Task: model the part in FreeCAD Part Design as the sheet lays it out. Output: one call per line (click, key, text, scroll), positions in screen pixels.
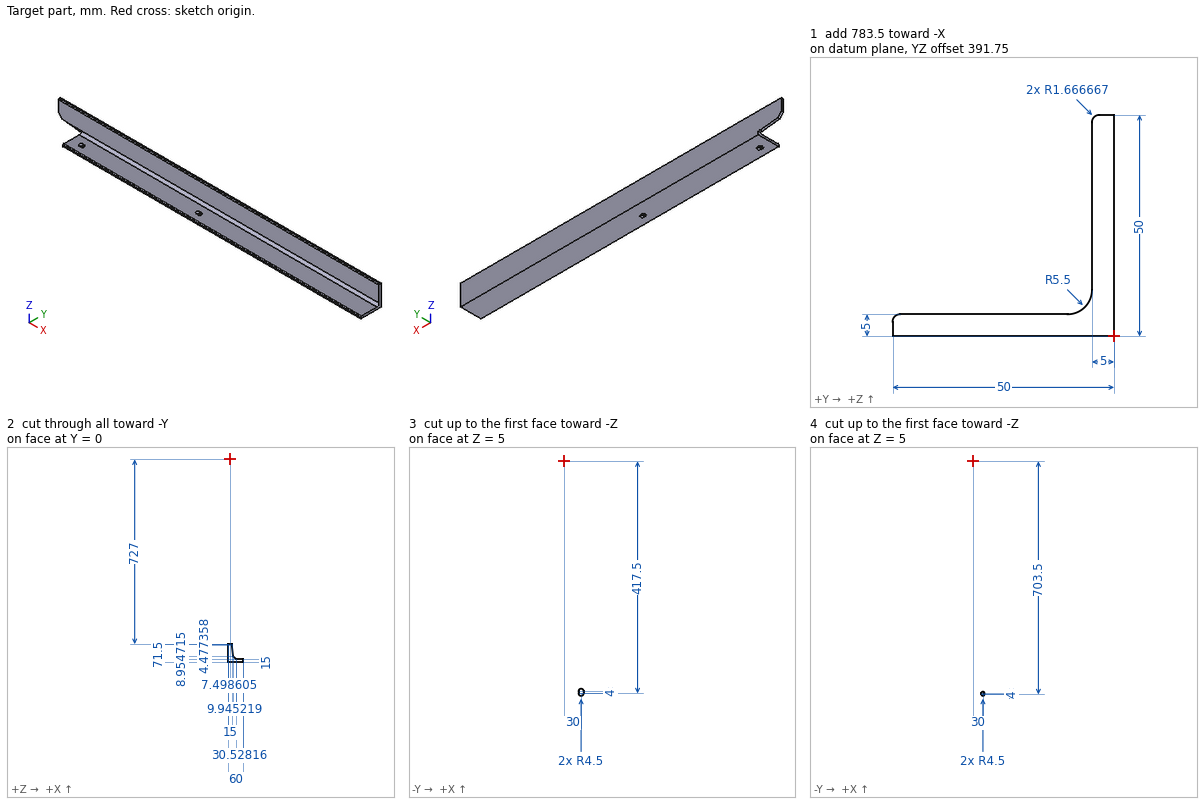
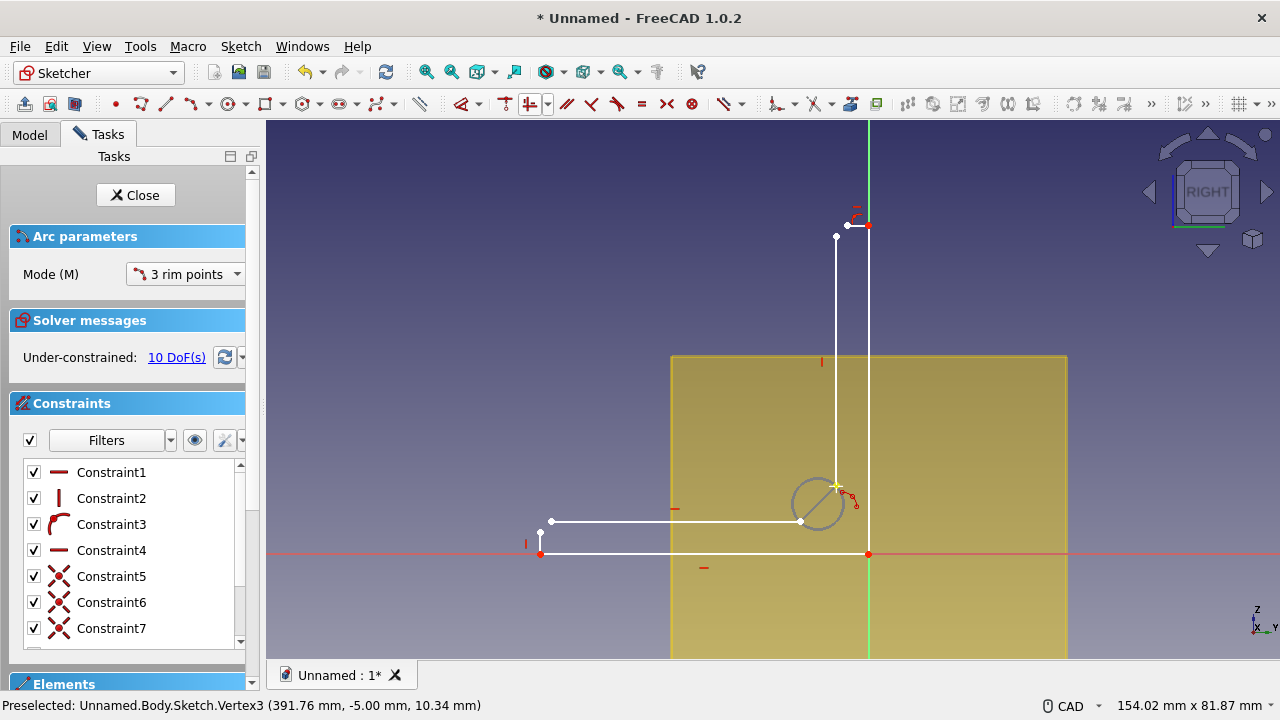
scroll(825, 511, up, 3)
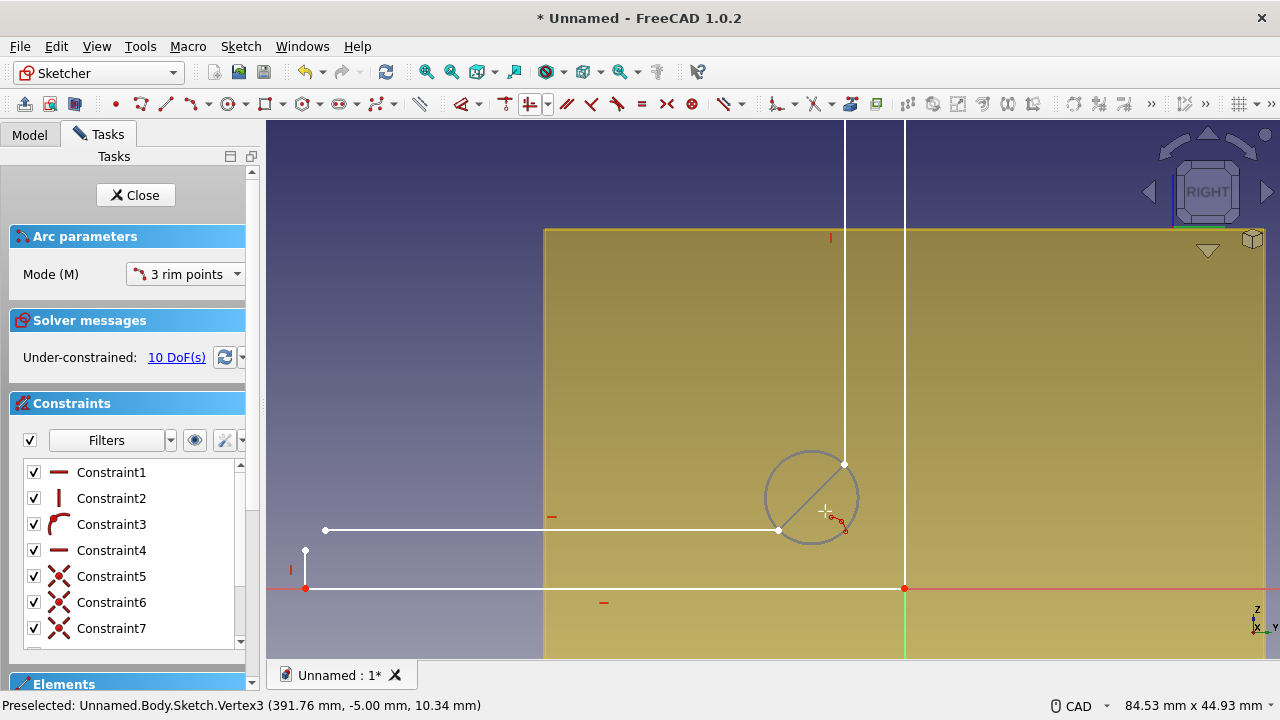
click(825, 510)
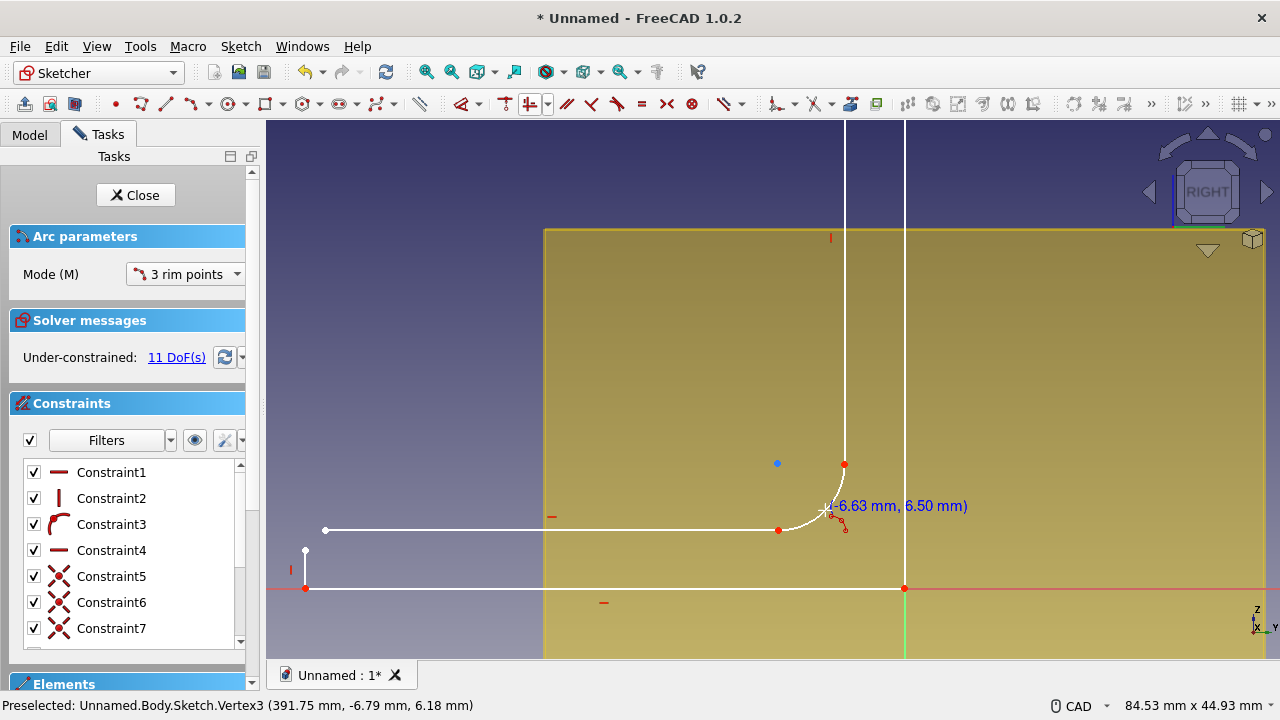
scroll(826, 512, down, 3)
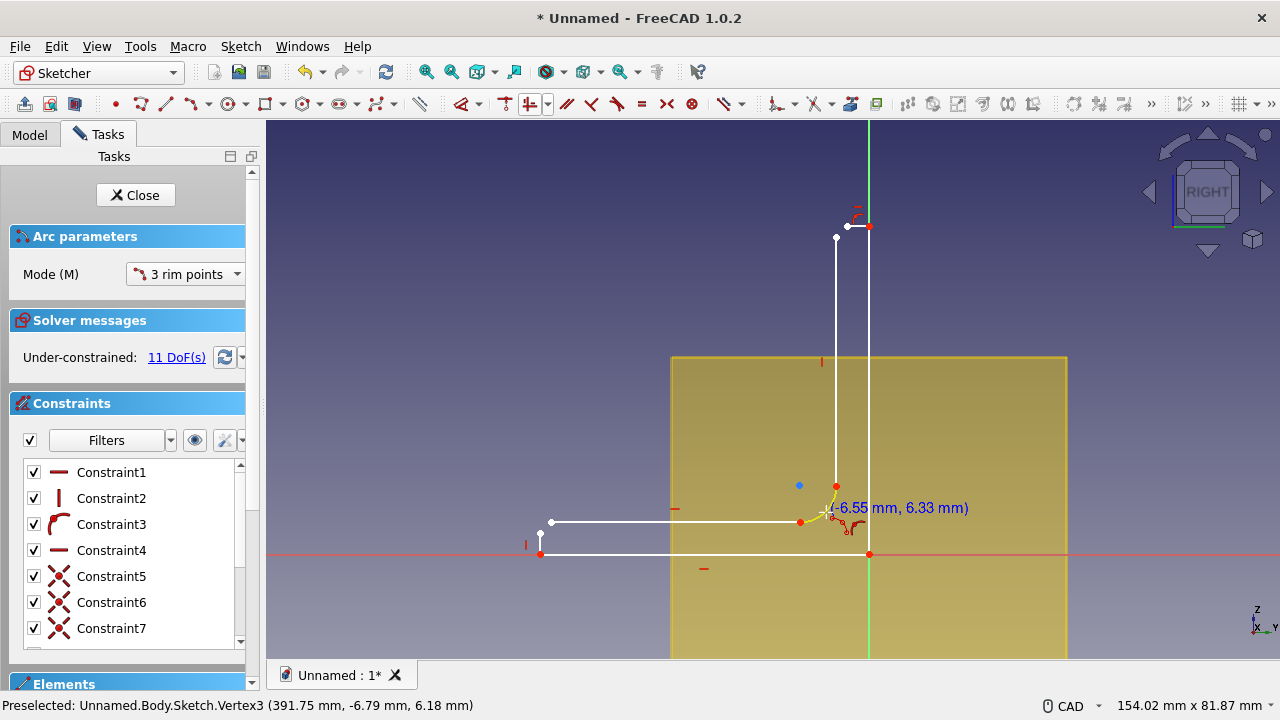
click(836, 237)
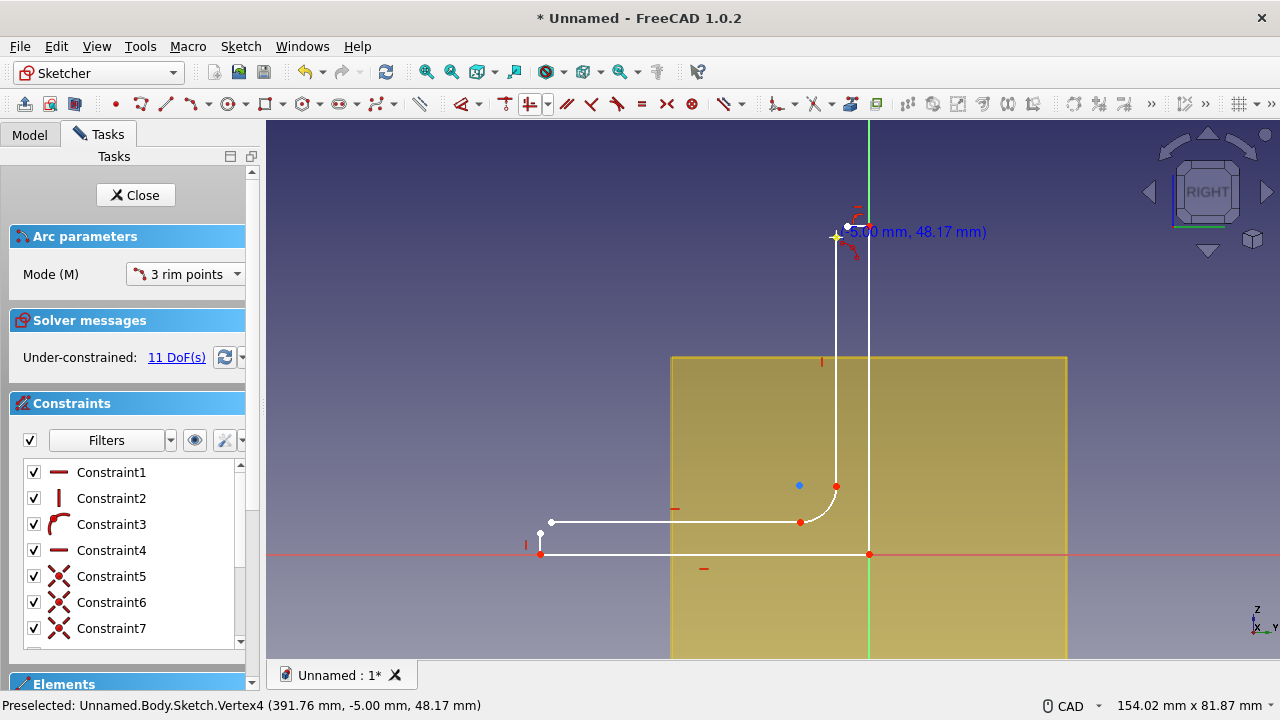
scroll(847, 225, up, 2)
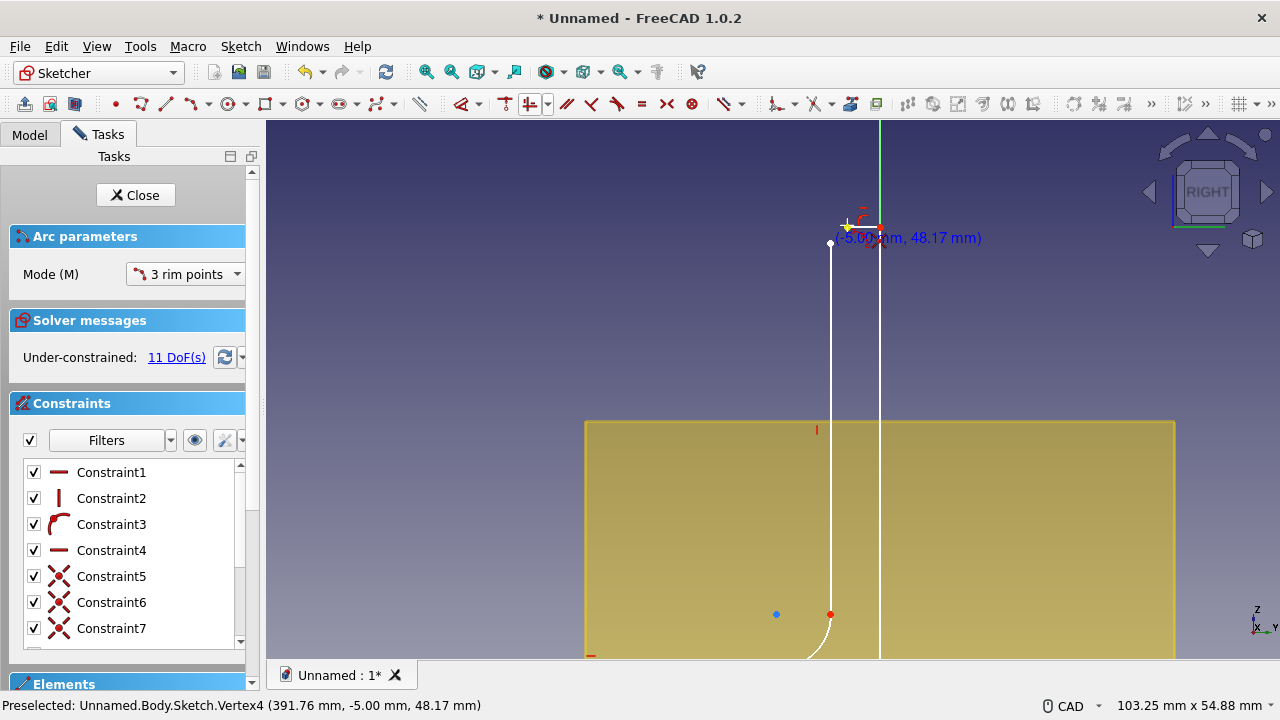
click(847, 227)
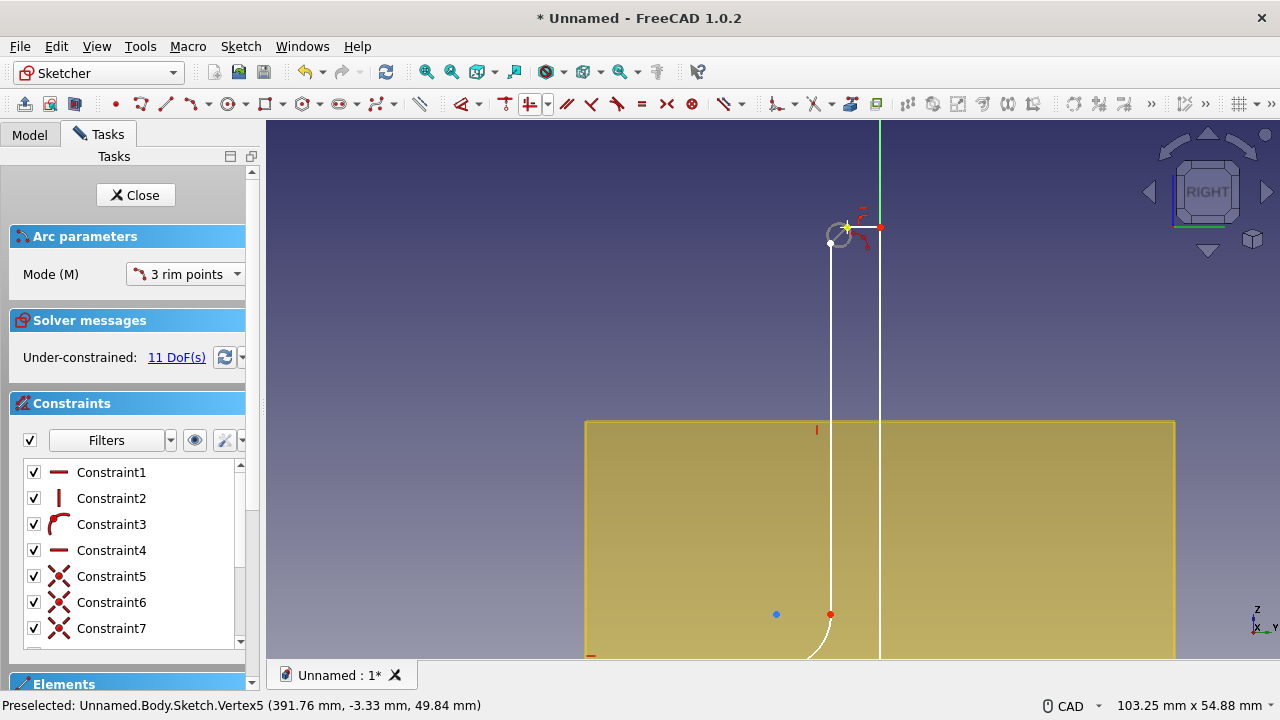
scroll(836, 230, up, 6)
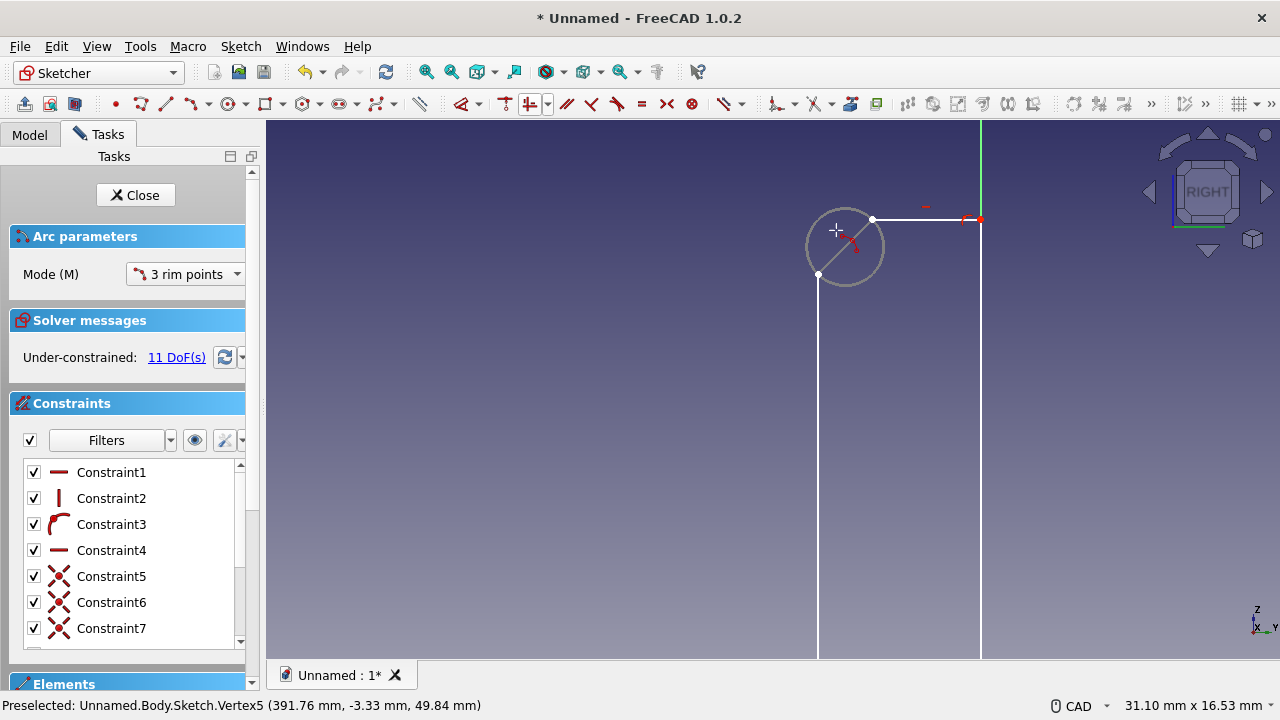
click(834, 230)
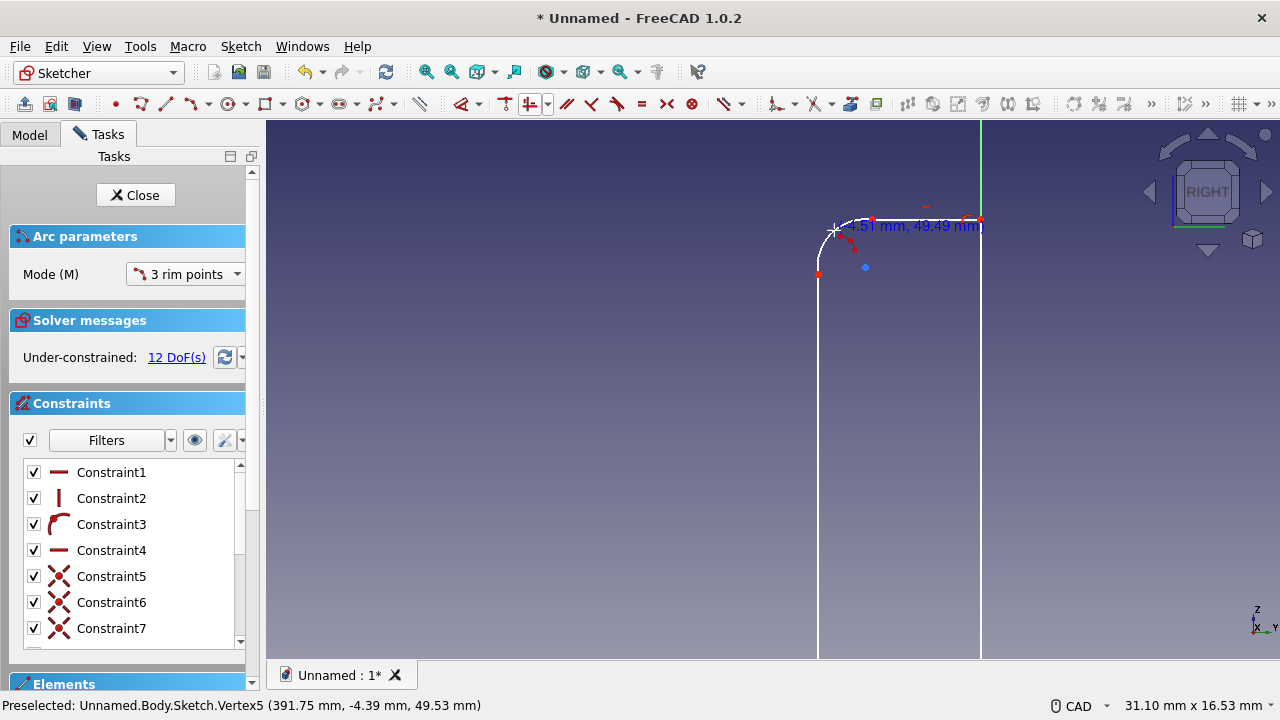
scroll(841, 228, down, 8)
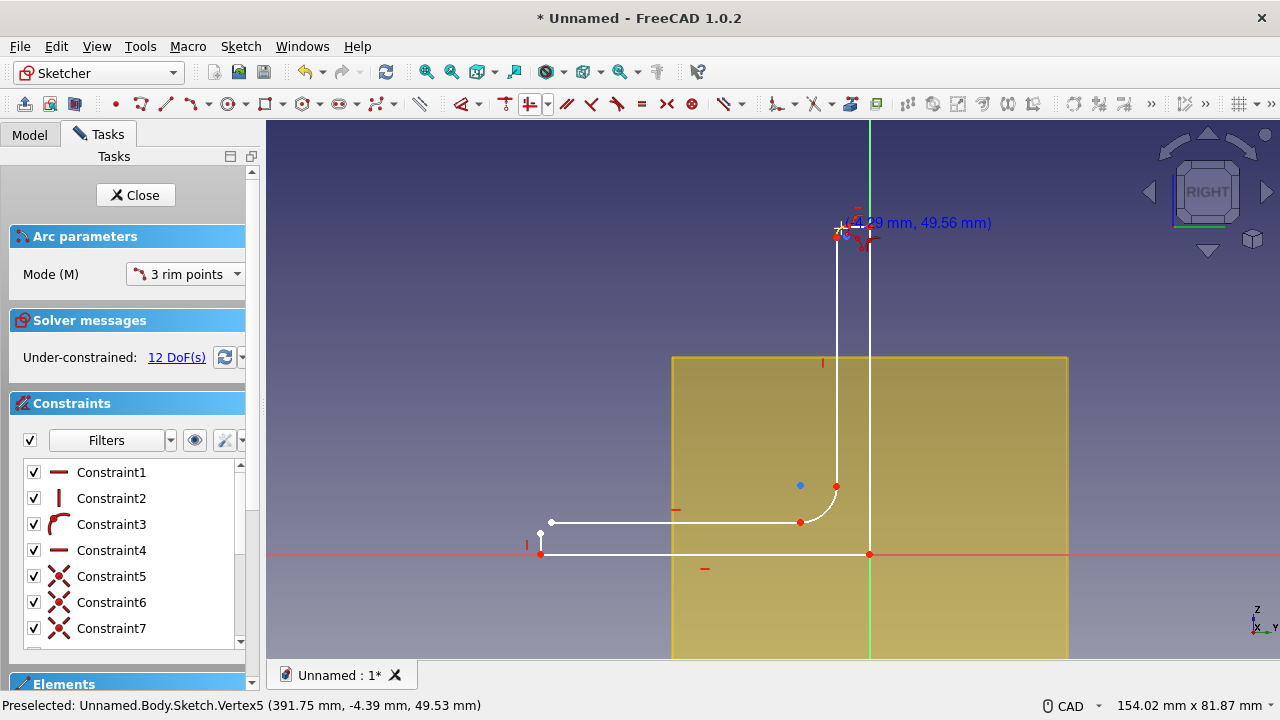
scroll(541, 533, up, 2)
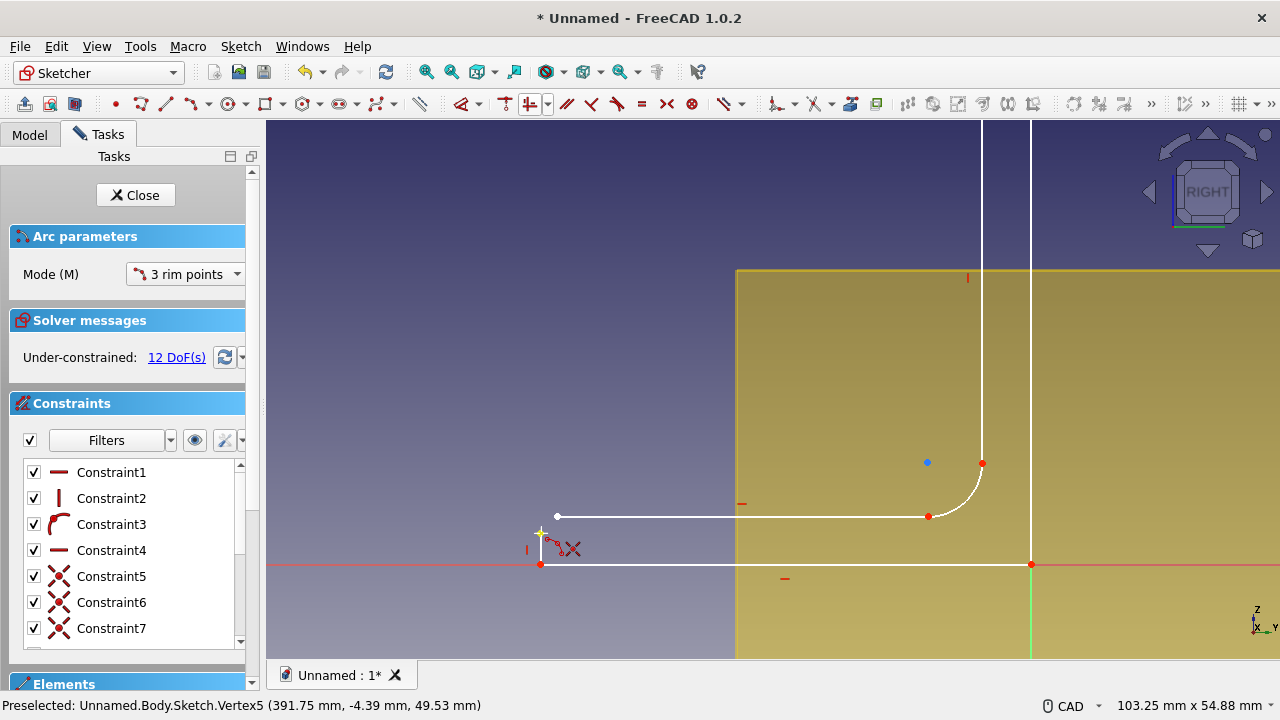
click(541, 533)
click(557, 517)